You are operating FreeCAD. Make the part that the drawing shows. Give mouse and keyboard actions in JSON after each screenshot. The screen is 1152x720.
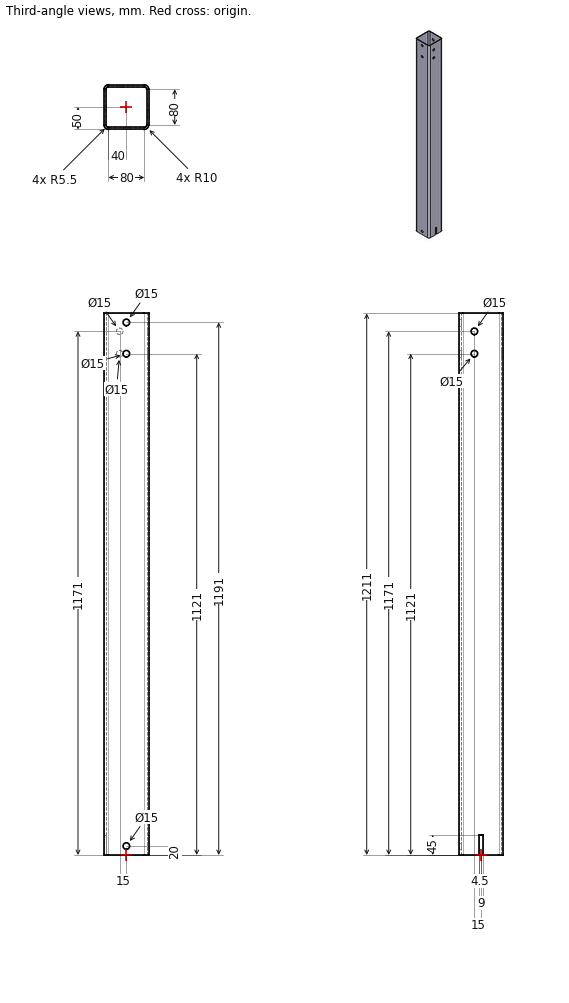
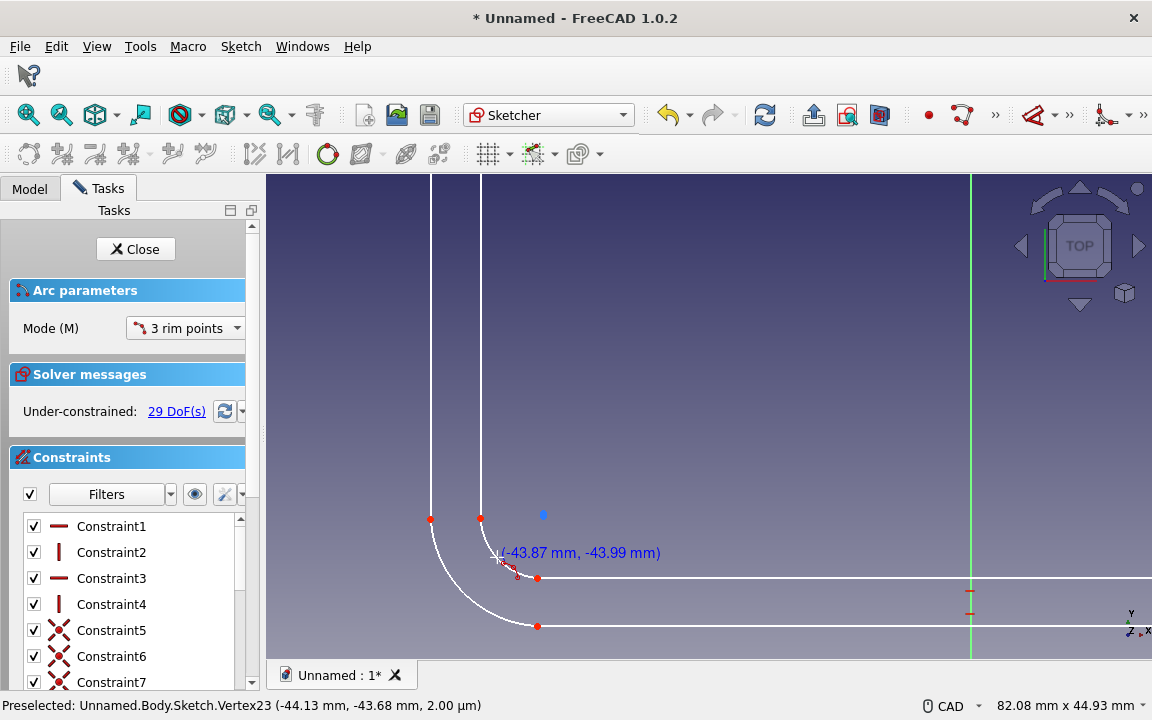
{"action": "scroll", "coordinate": [498, 560], "scroll_direction": "down", "scroll_amount": 6}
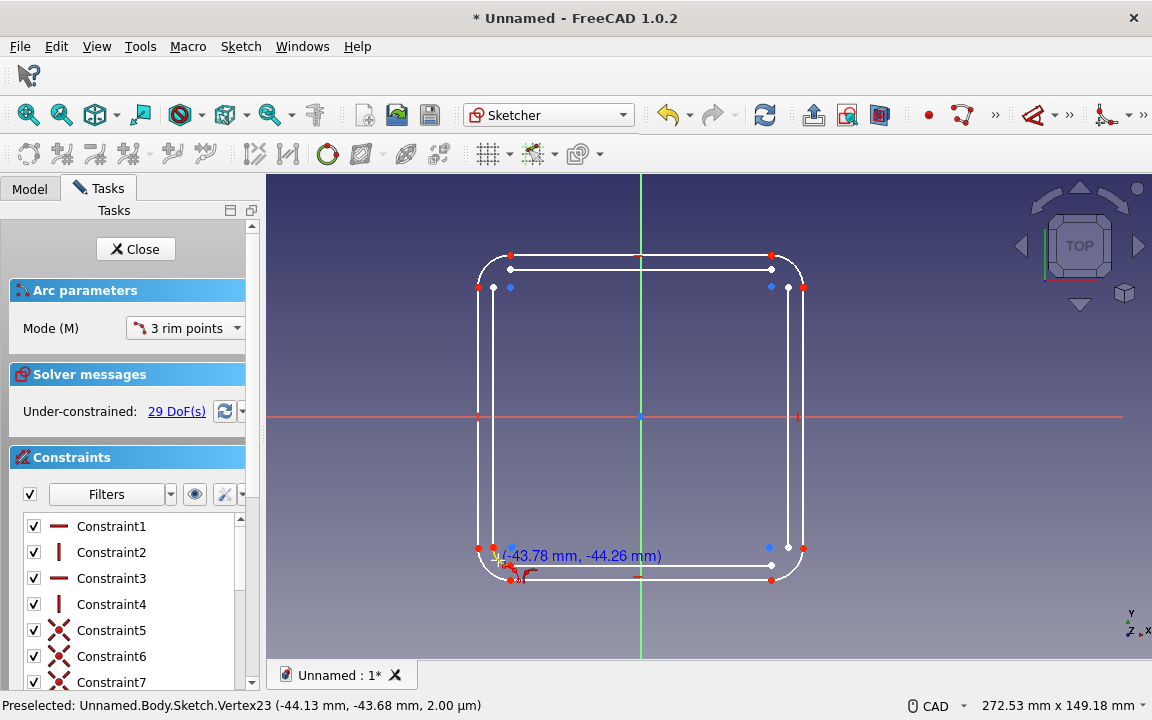
{"action": "left_click", "coordinate": [493, 288]}
{"action": "left_click", "coordinate": [510, 270]}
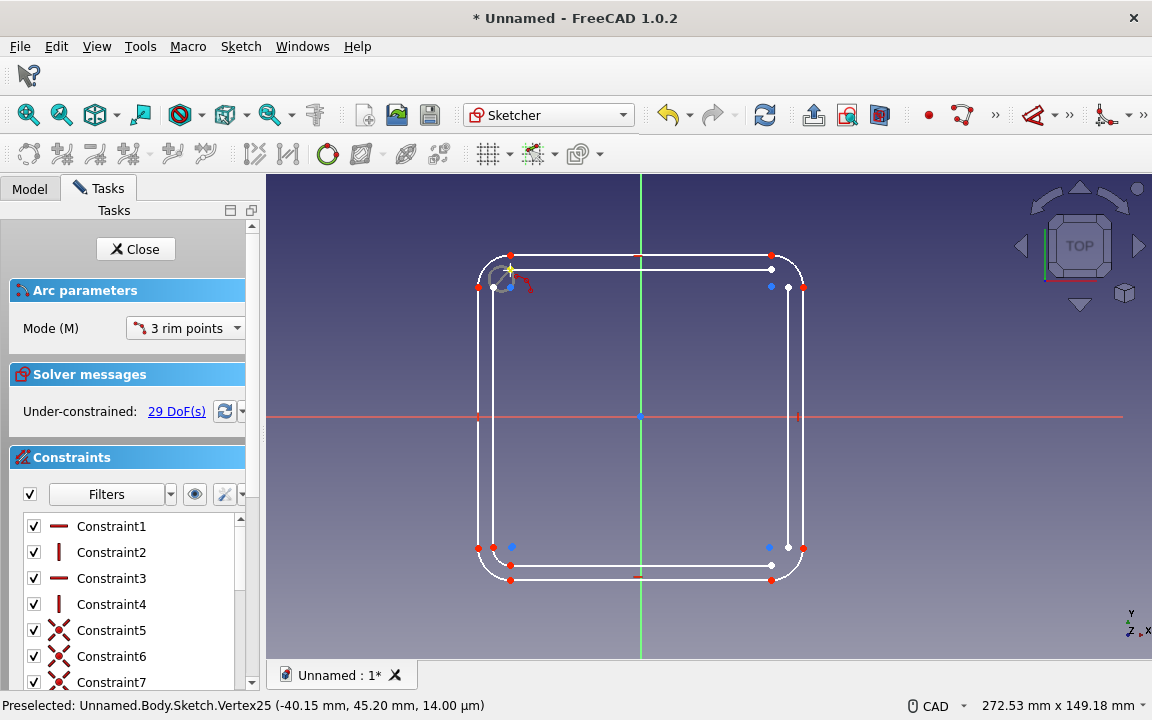
{"action": "scroll", "coordinate": [498, 274], "scroll_direction": "up", "scroll_amount": 6}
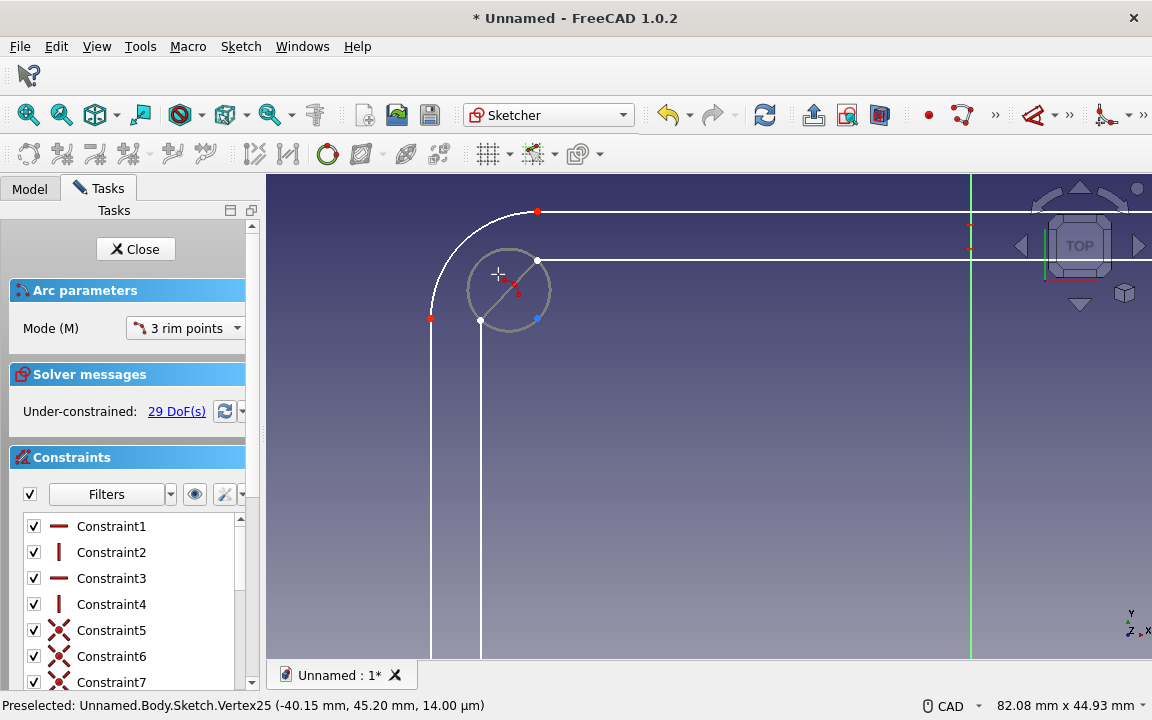
{"action": "left_click", "coordinate": [497, 274]}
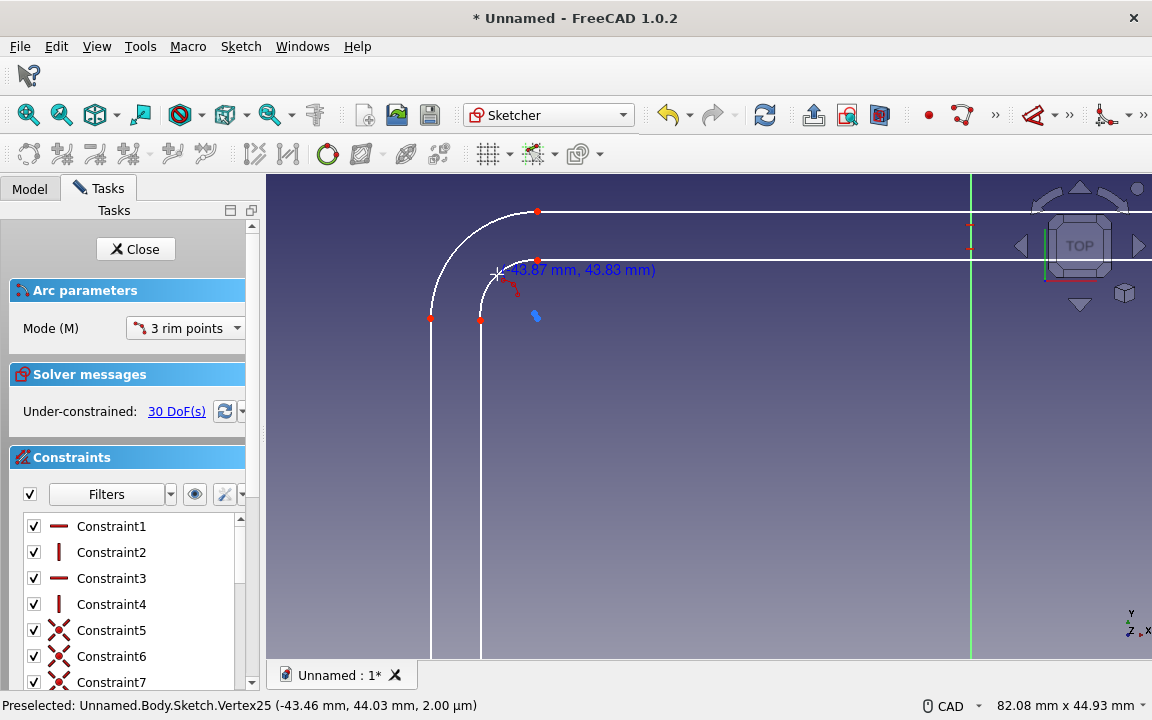
{"action": "scroll", "coordinate": [498, 274], "scroll_direction": "down", "scroll_amount": 6}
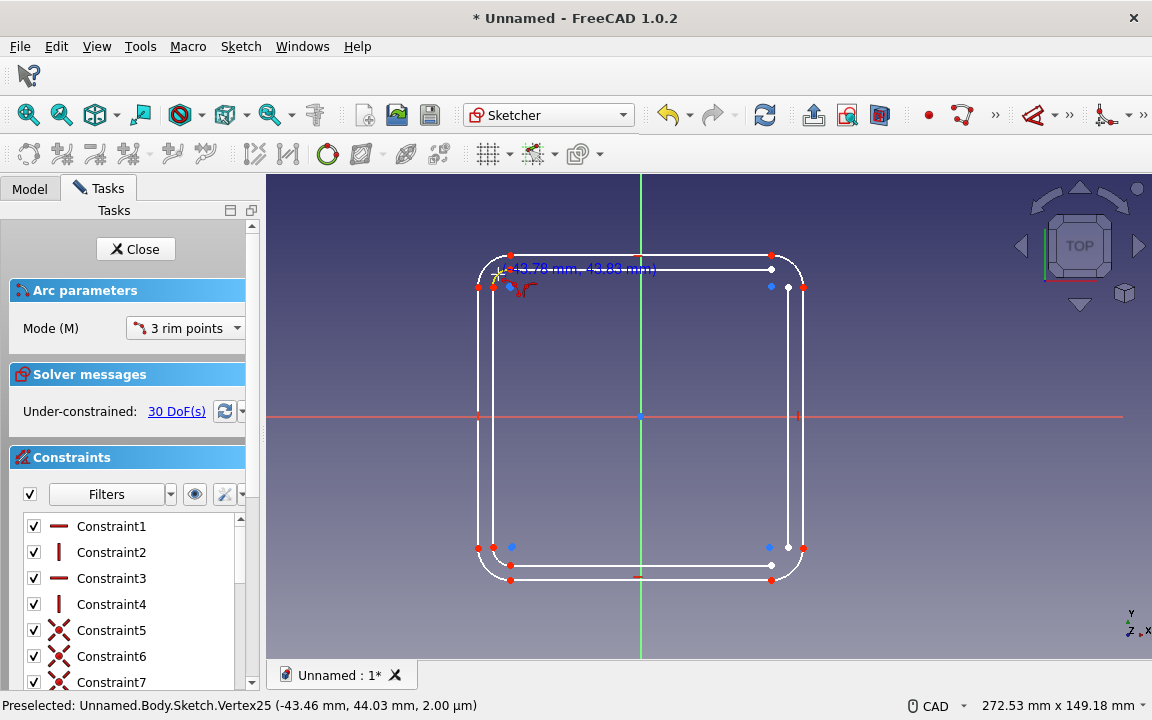
{"action": "left_click", "coordinate": [771, 270]}
{"action": "left_click", "coordinate": [788, 288]}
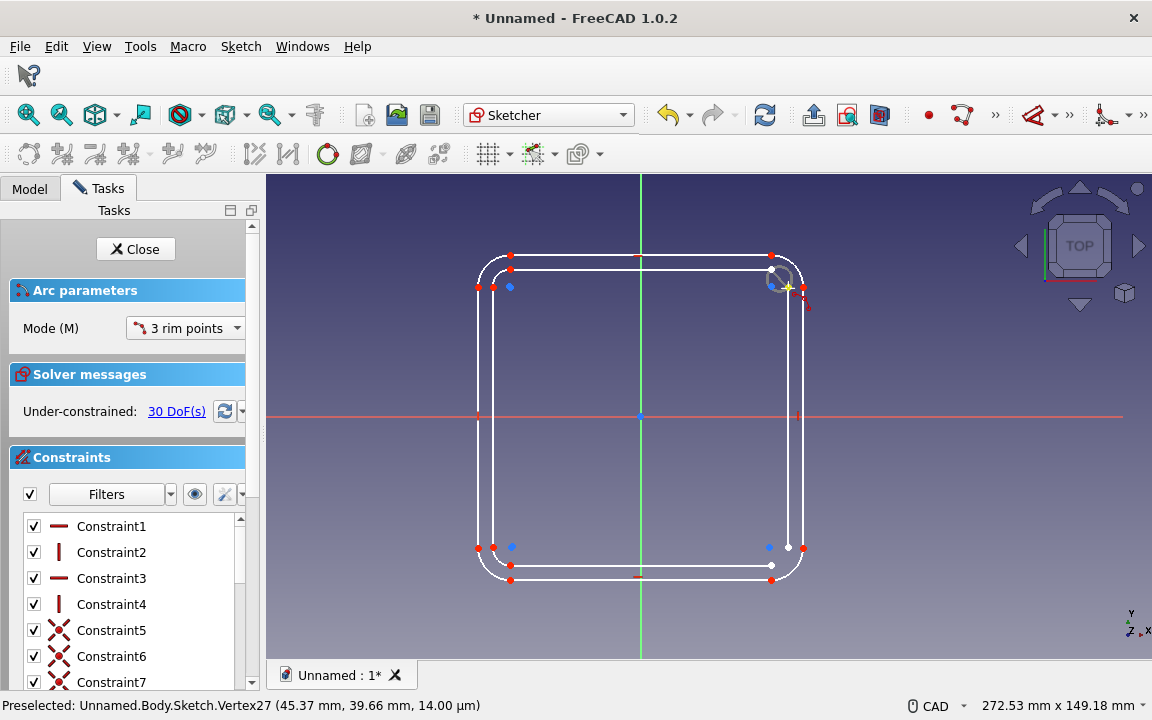
{"action": "scroll", "coordinate": [783, 274], "scroll_direction": "up", "scroll_amount": 6}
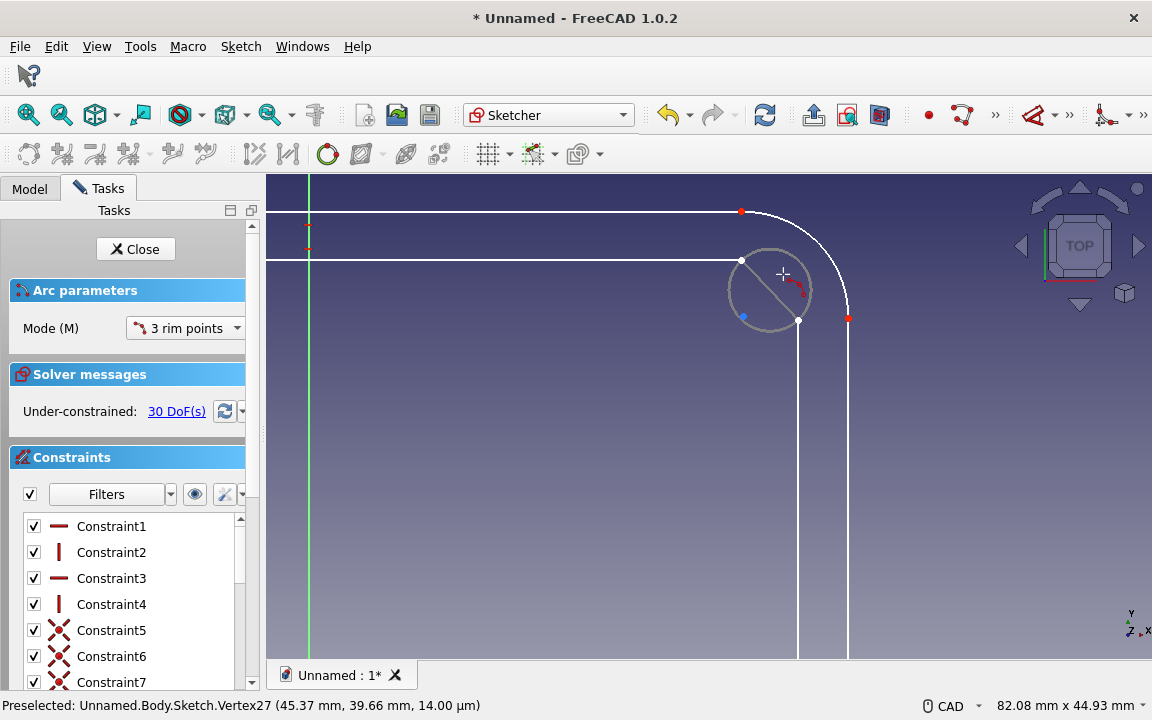
{"action": "left_click", "coordinate": [782, 274]}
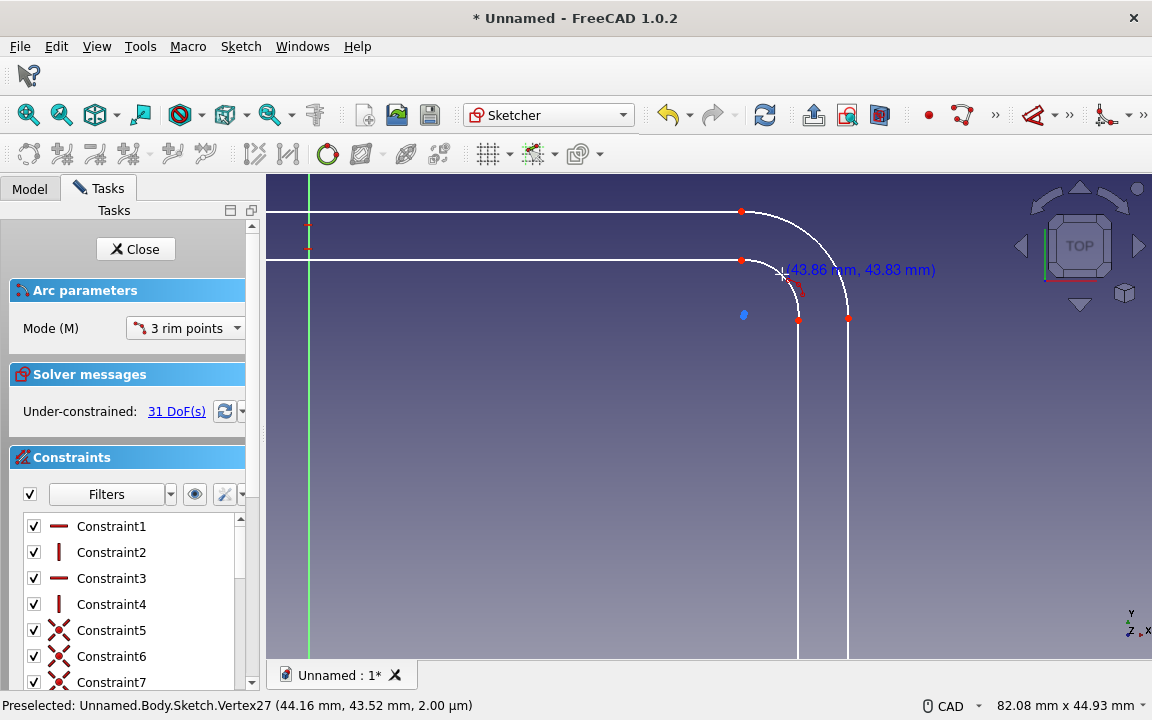
{"action": "scroll", "coordinate": [784, 274], "scroll_direction": "down", "scroll_amount": 6}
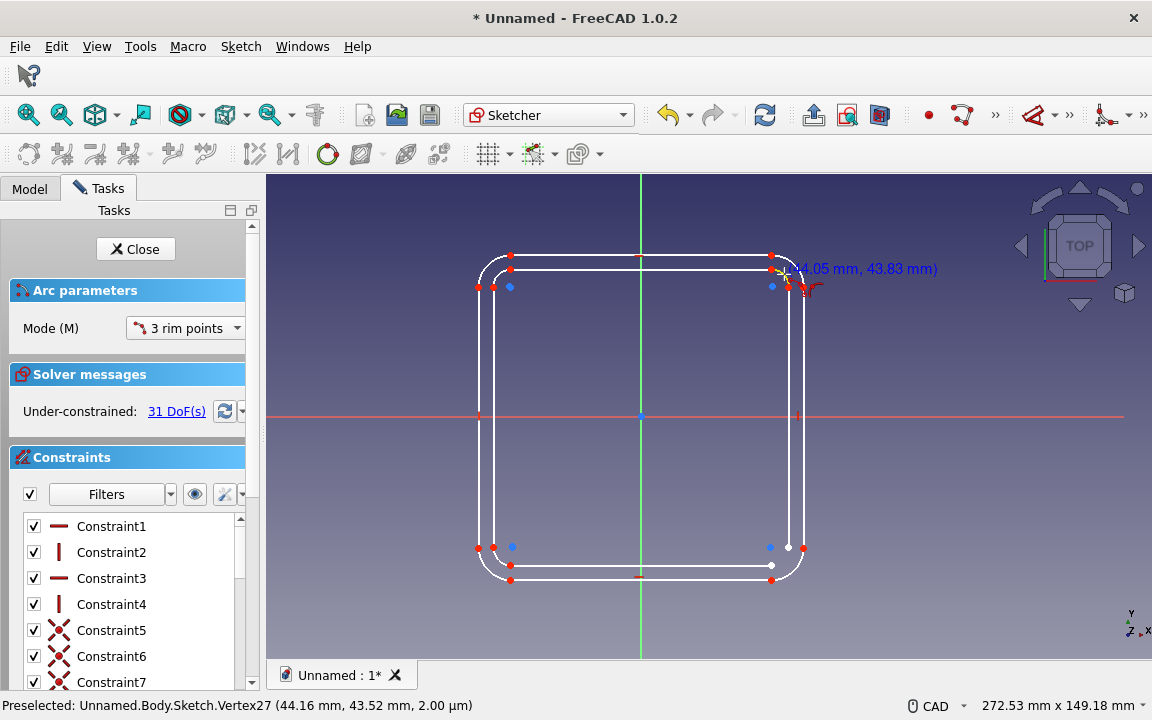
{"action": "left_click", "coordinate": [789, 548]}
{"action": "left_click", "coordinate": [772, 566]}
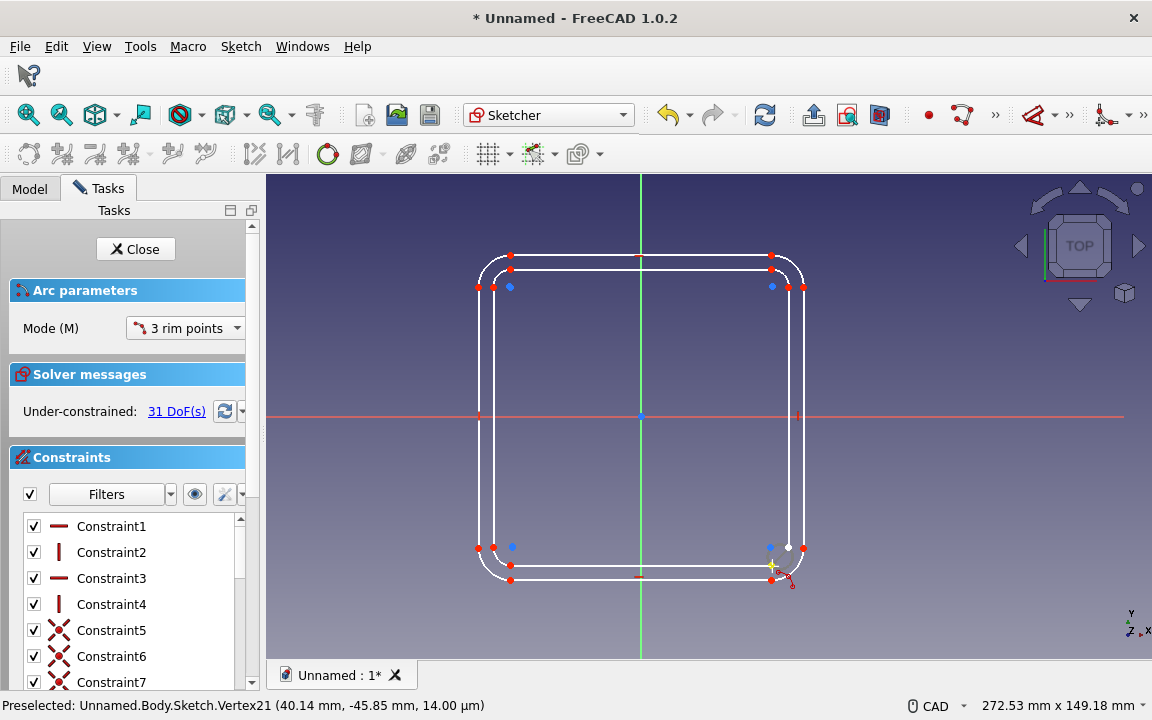
{"action": "scroll", "coordinate": [784, 560], "scroll_direction": "up", "scroll_amount": 6}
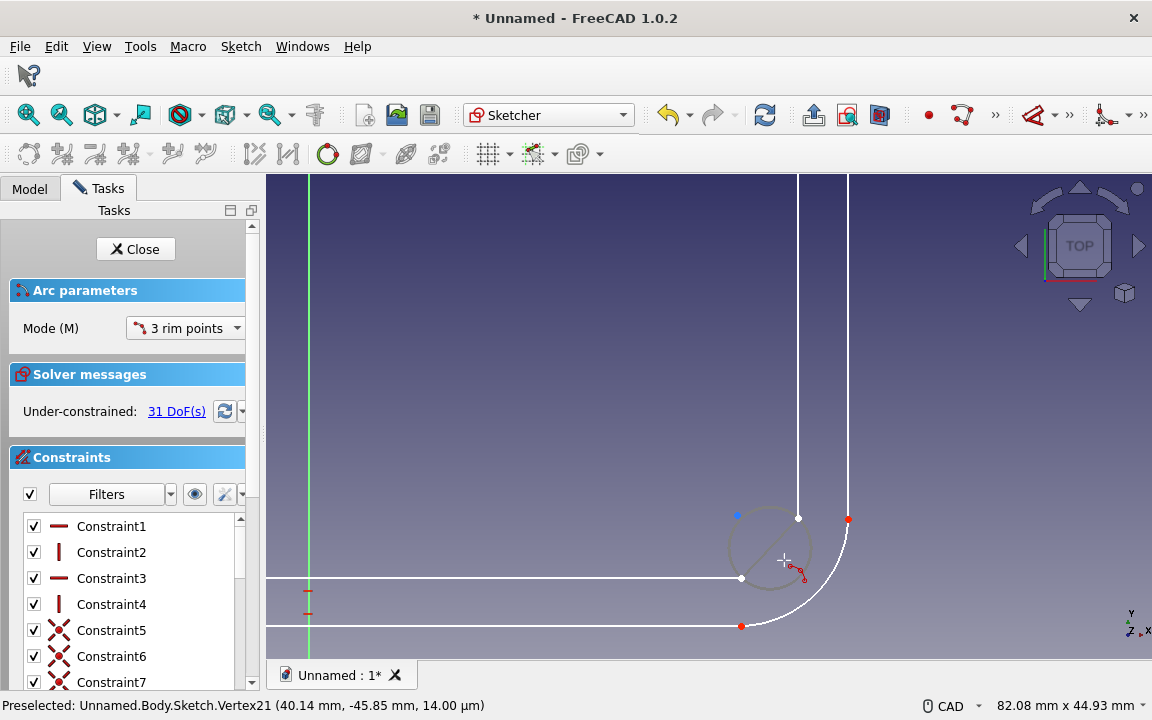
{"action": "left_click", "coordinate": [782, 557]}
{"action": "key", "text": "Escape"}